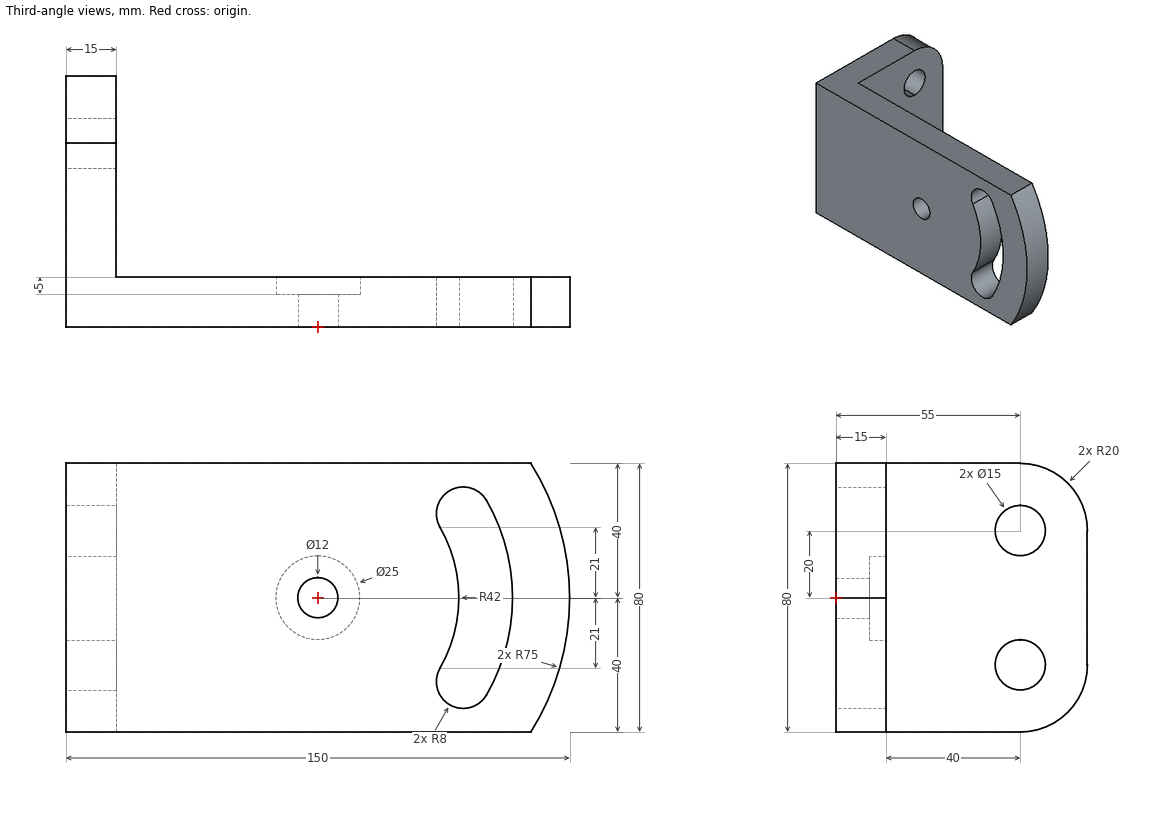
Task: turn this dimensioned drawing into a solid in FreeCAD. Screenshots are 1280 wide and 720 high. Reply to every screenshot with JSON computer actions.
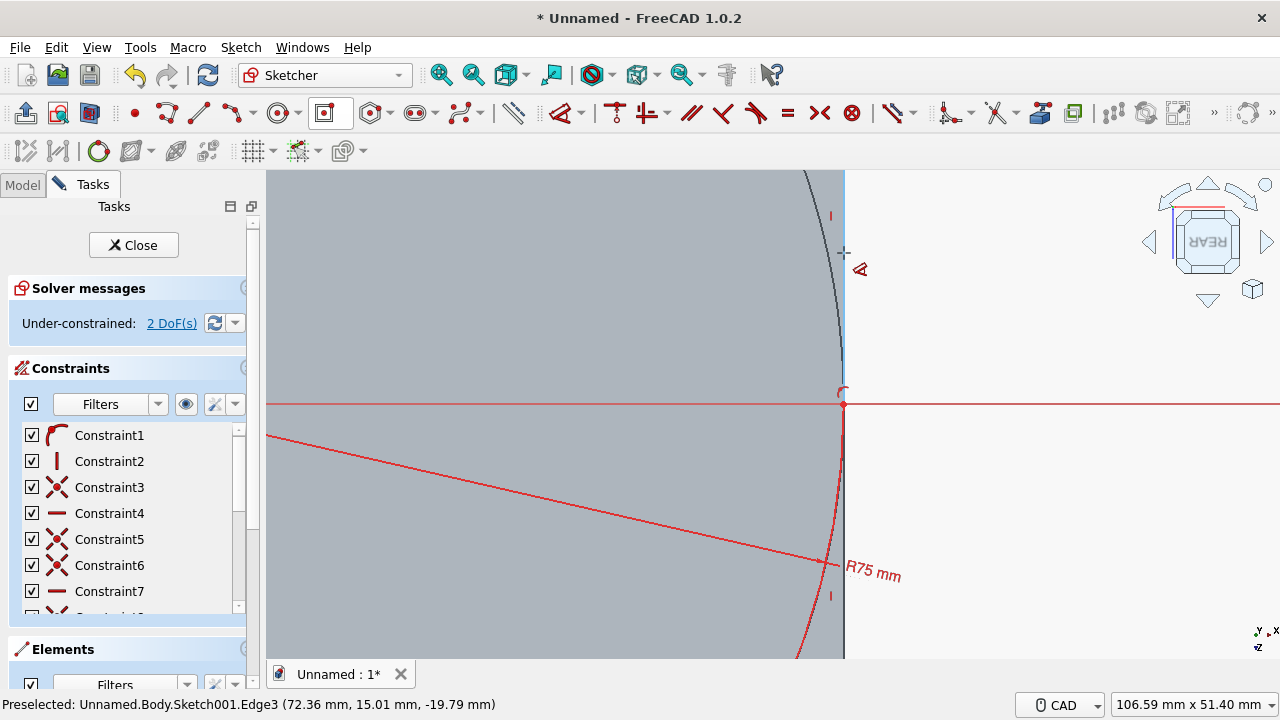
{"action": "left_click", "coordinate": [844, 253]}
{"action": "left_click", "coordinate": [878, 301]}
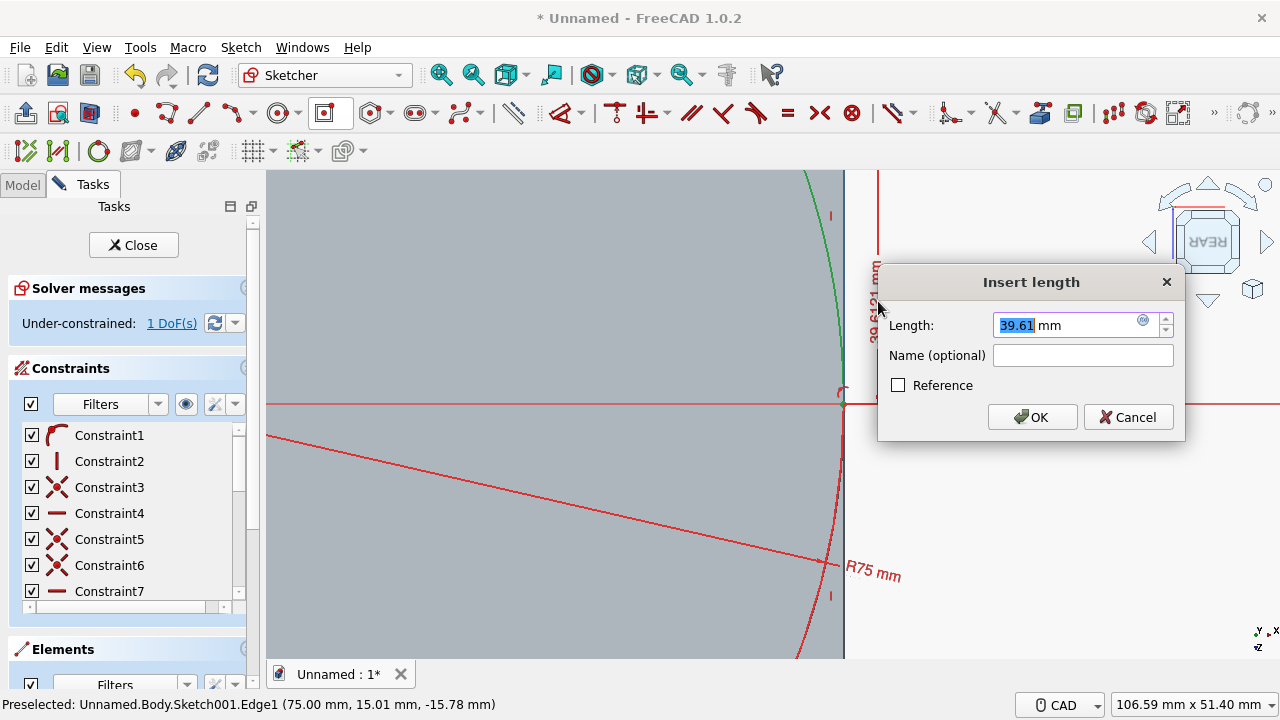
{"action": "type", "text": "40"}
{"action": "key", "text": "Return"}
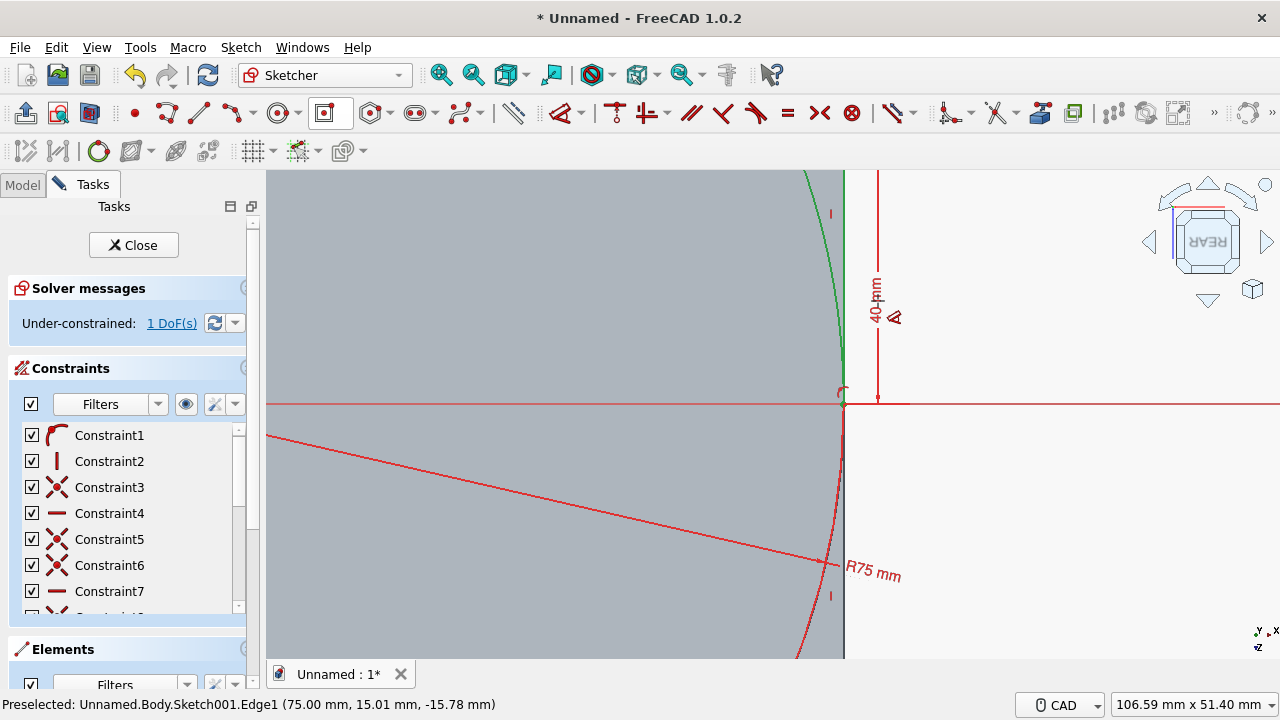
{"action": "scroll", "coordinate": [844, 519], "scroll_direction": "up", "scroll_amount": 3}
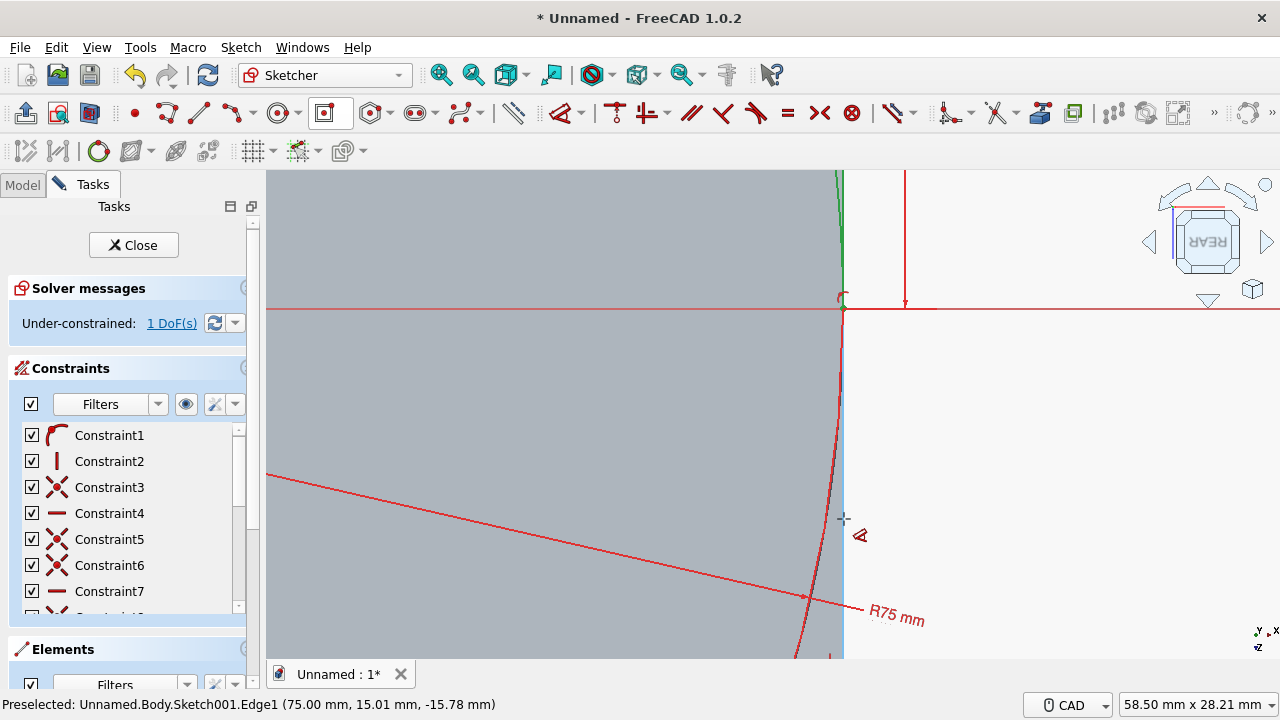
{"action": "left_click", "coordinate": [843, 518]}
{"action": "left_click", "coordinate": [877, 470]}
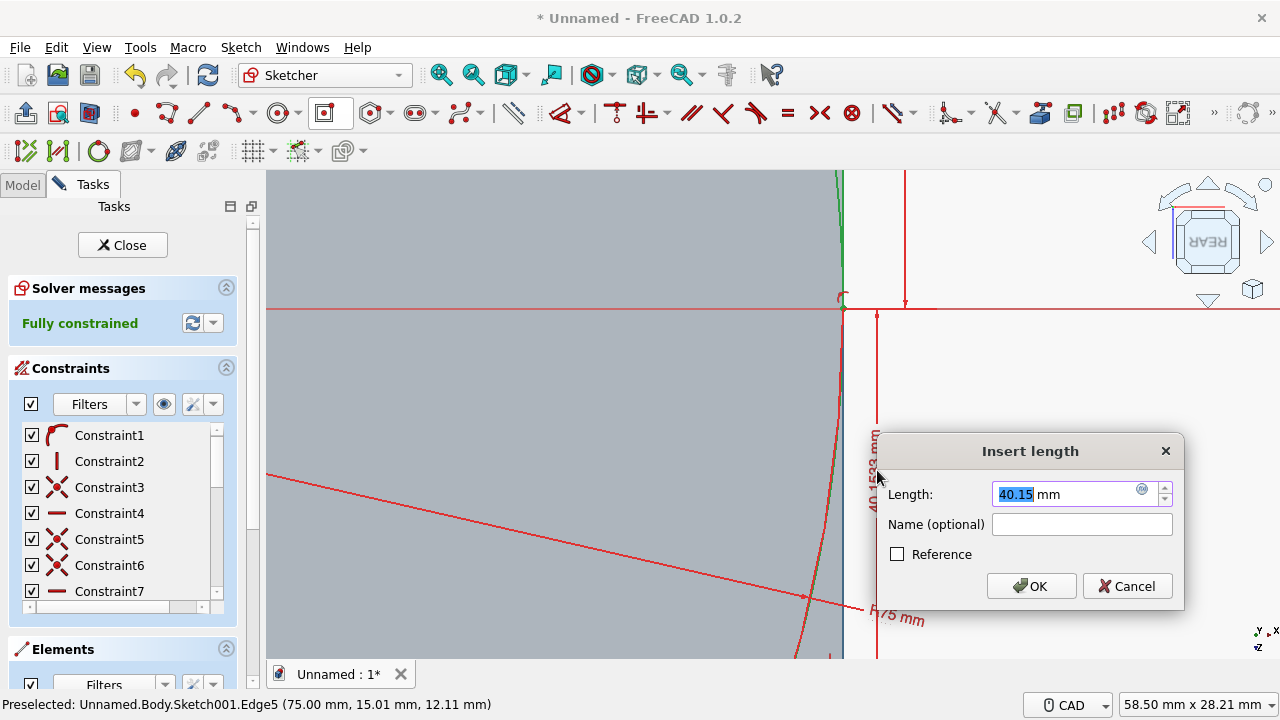
{"action": "type", "text": "40"}
{"action": "key", "text": "Return"}
{"action": "key", "text": "Escape"}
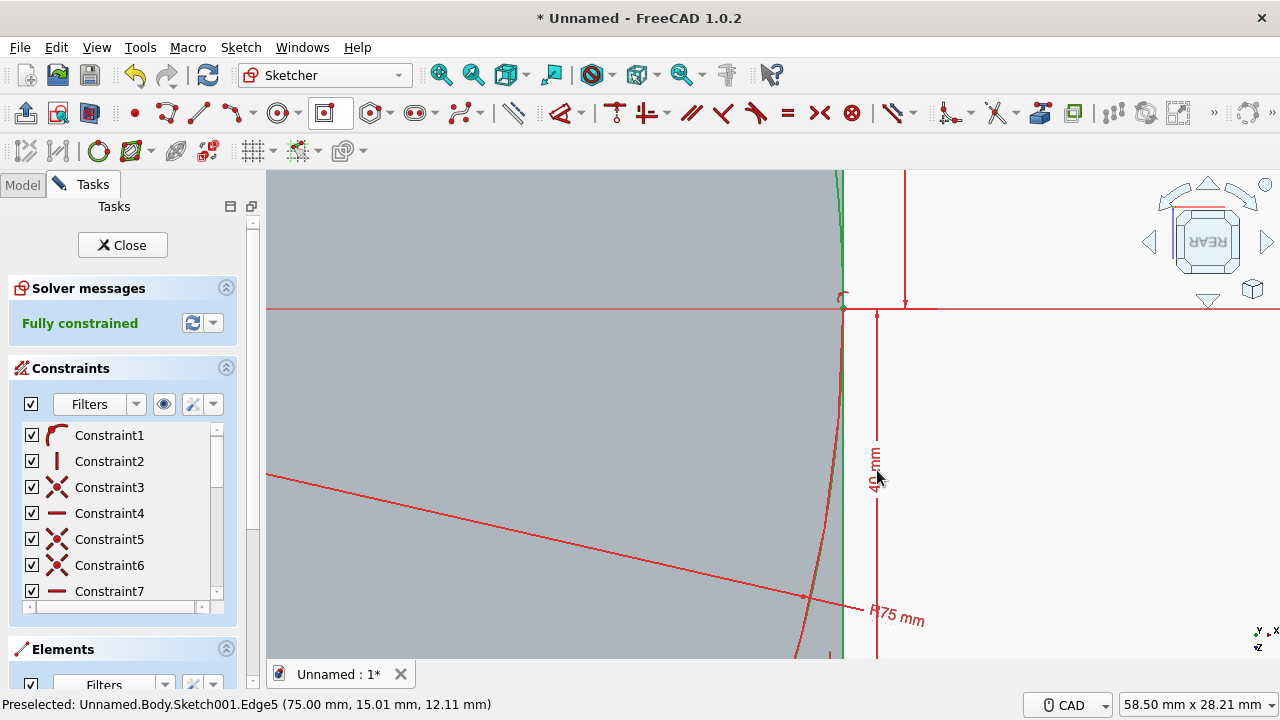
{"action": "left_click", "coordinate": [123, 245]}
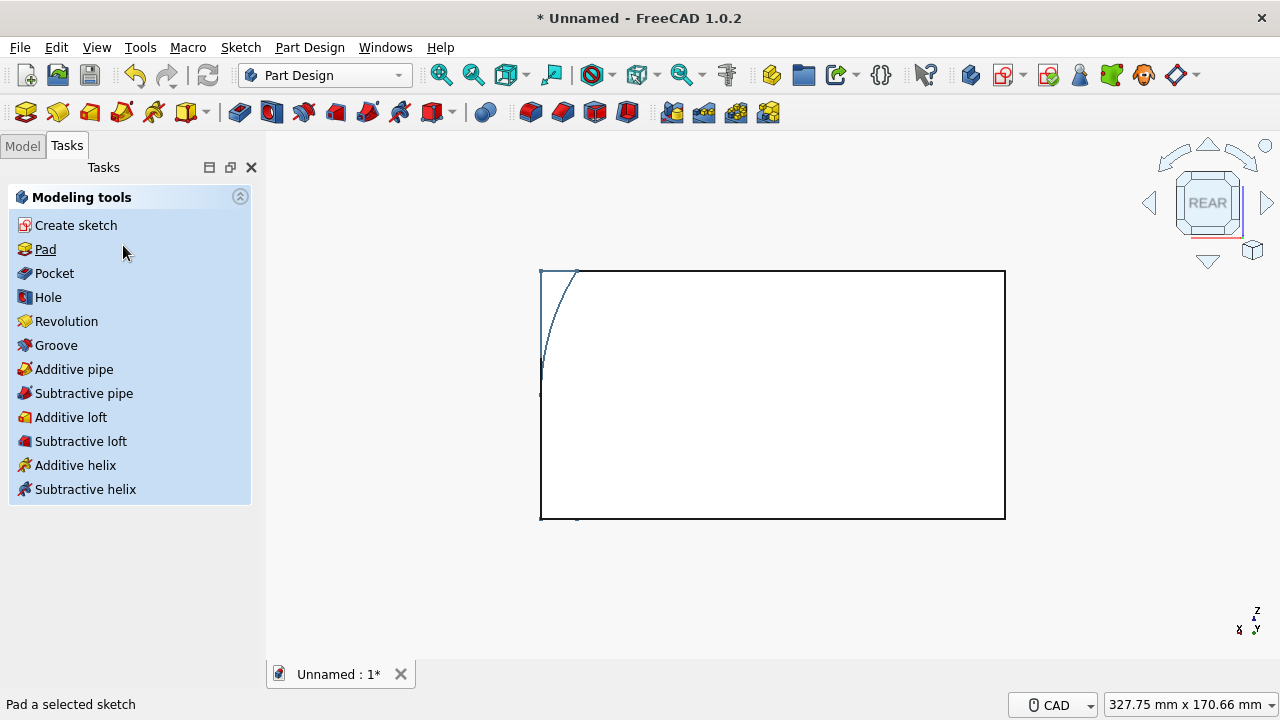
{"action": "left_click", "coordinate": [240, 112]}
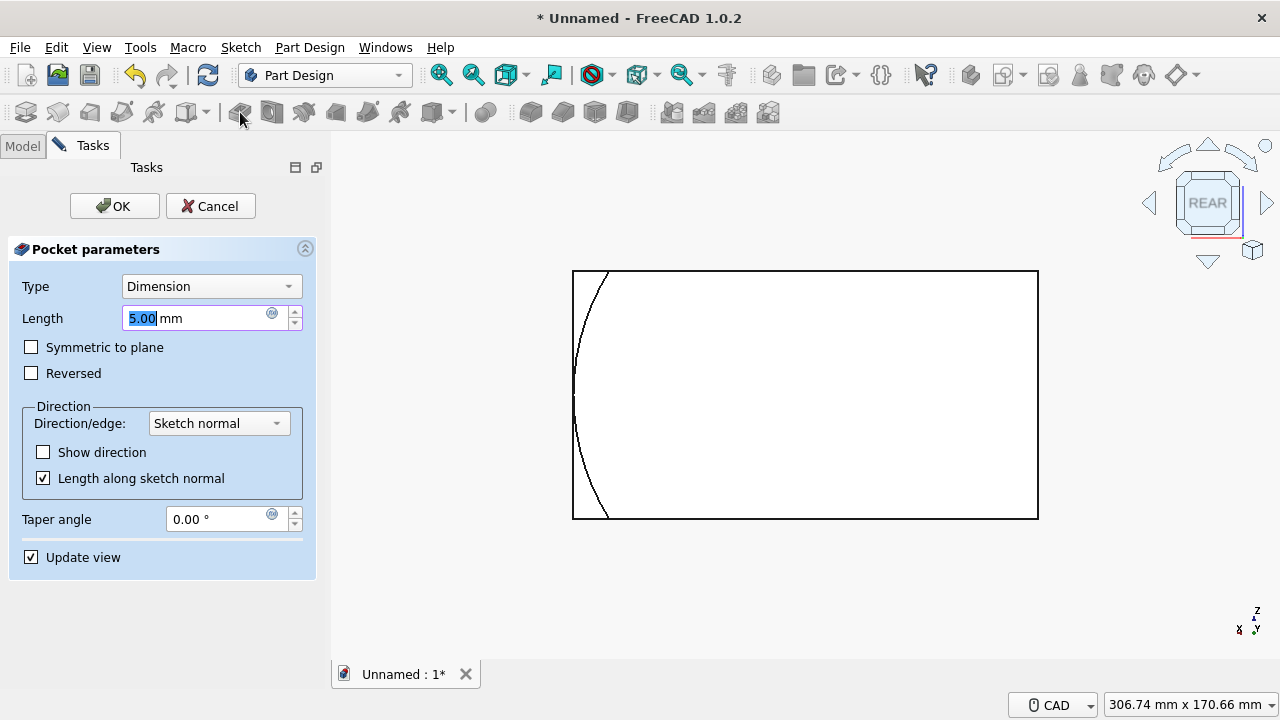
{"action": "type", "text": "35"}
{"action": "key", "text": "Tab"}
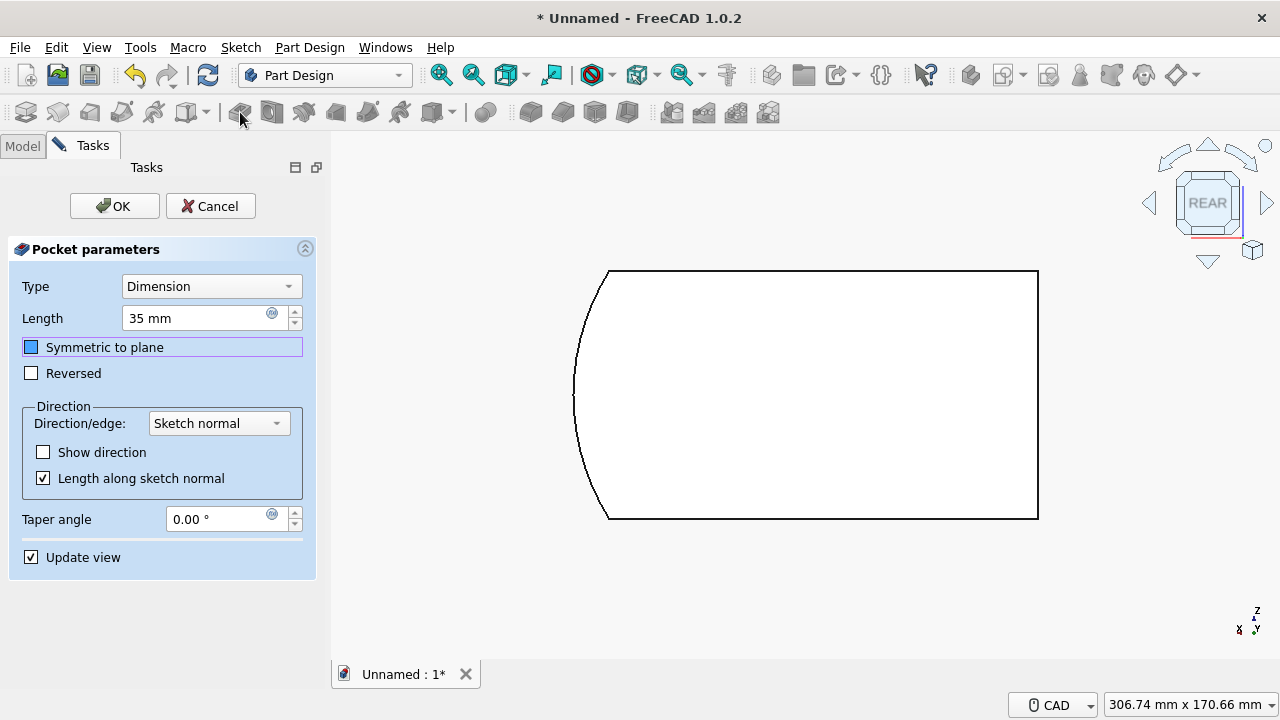
{"action": "left_click", "coordinate": [115, 206]}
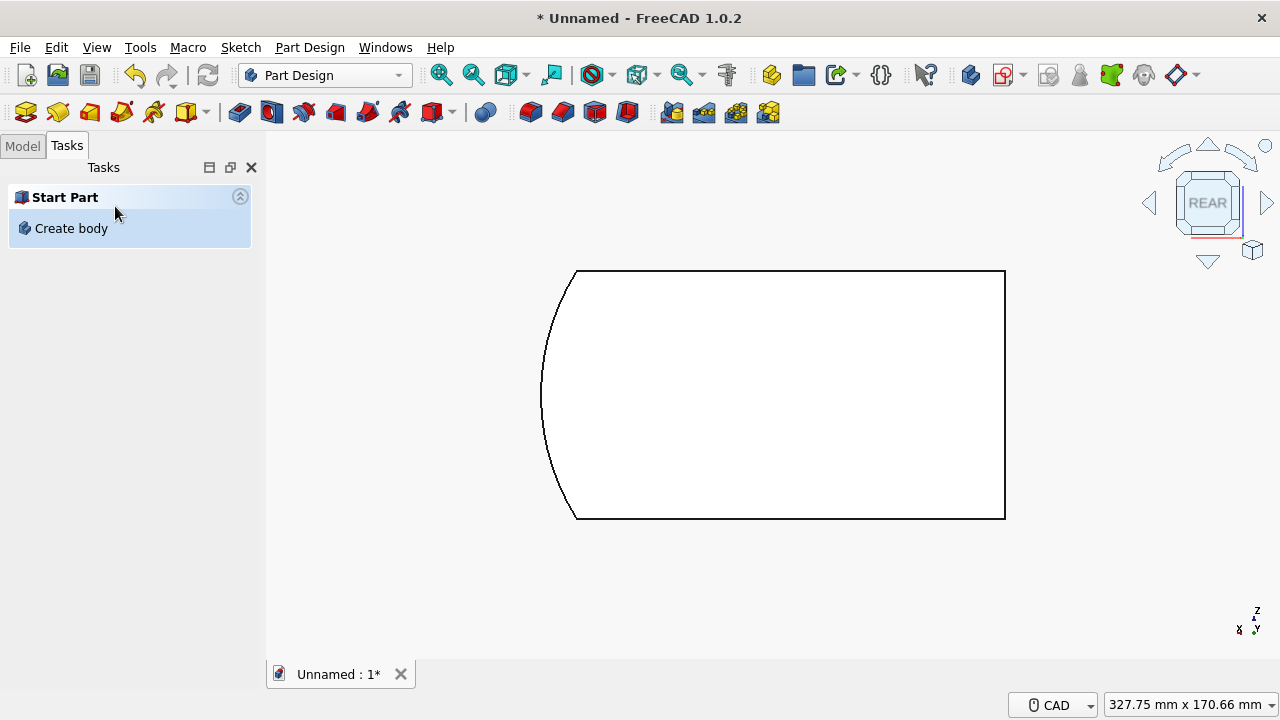
{"action": "left_click", "coordinate": [707, 394]}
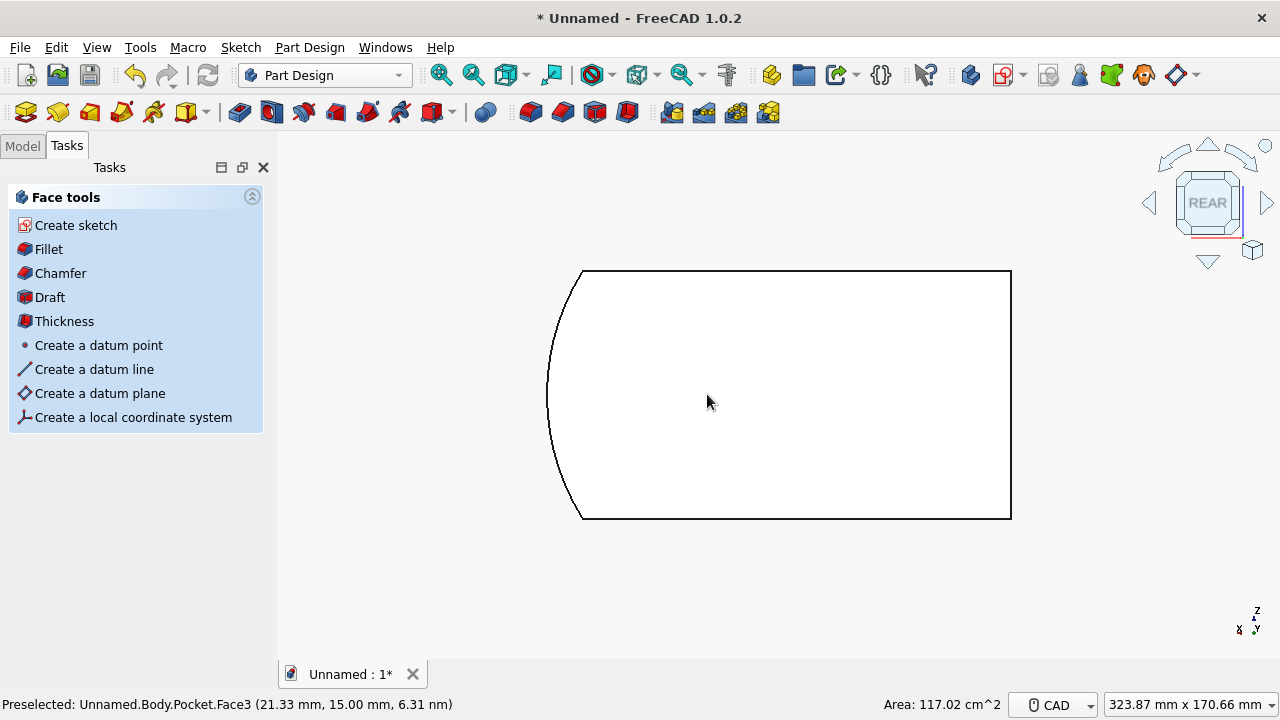
{"action": "left_click", "coordinate": [1004, 76]}